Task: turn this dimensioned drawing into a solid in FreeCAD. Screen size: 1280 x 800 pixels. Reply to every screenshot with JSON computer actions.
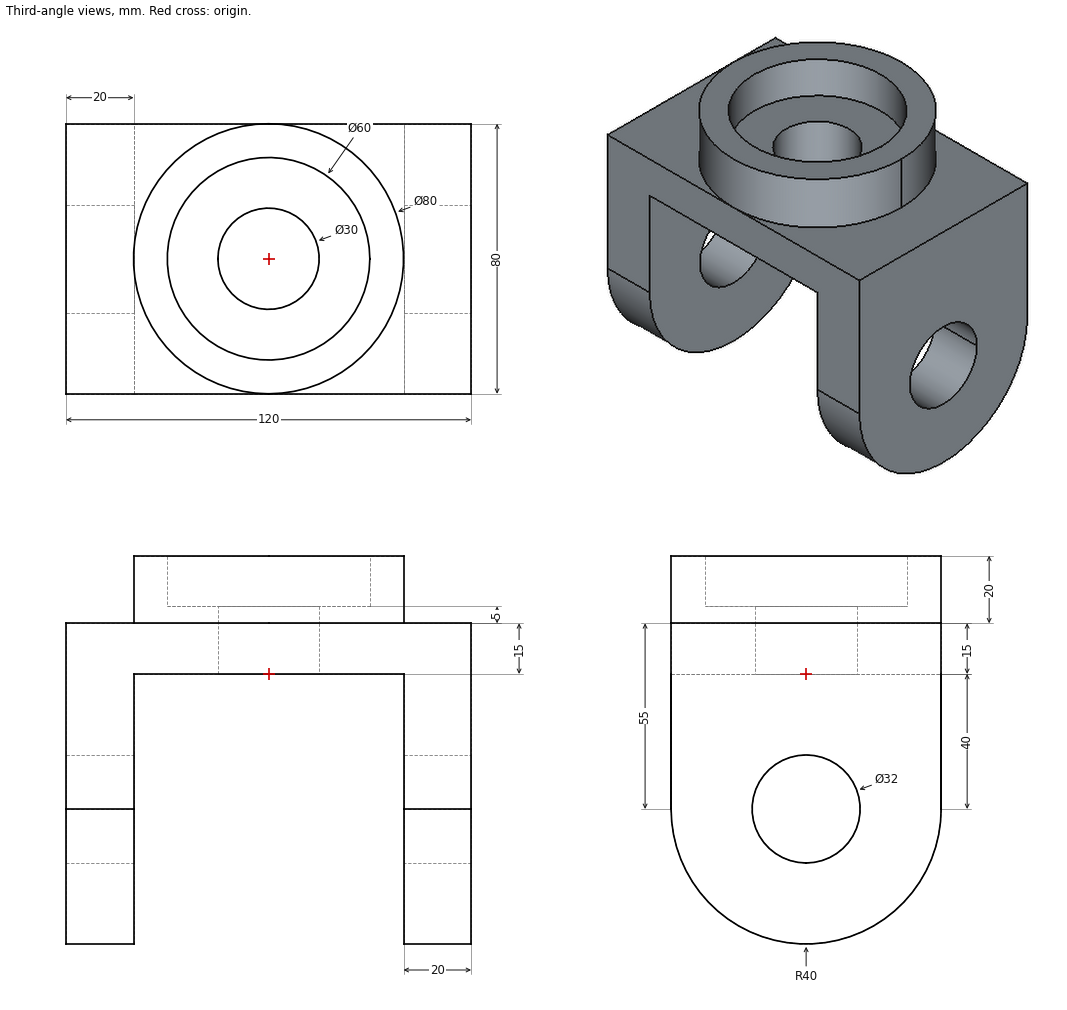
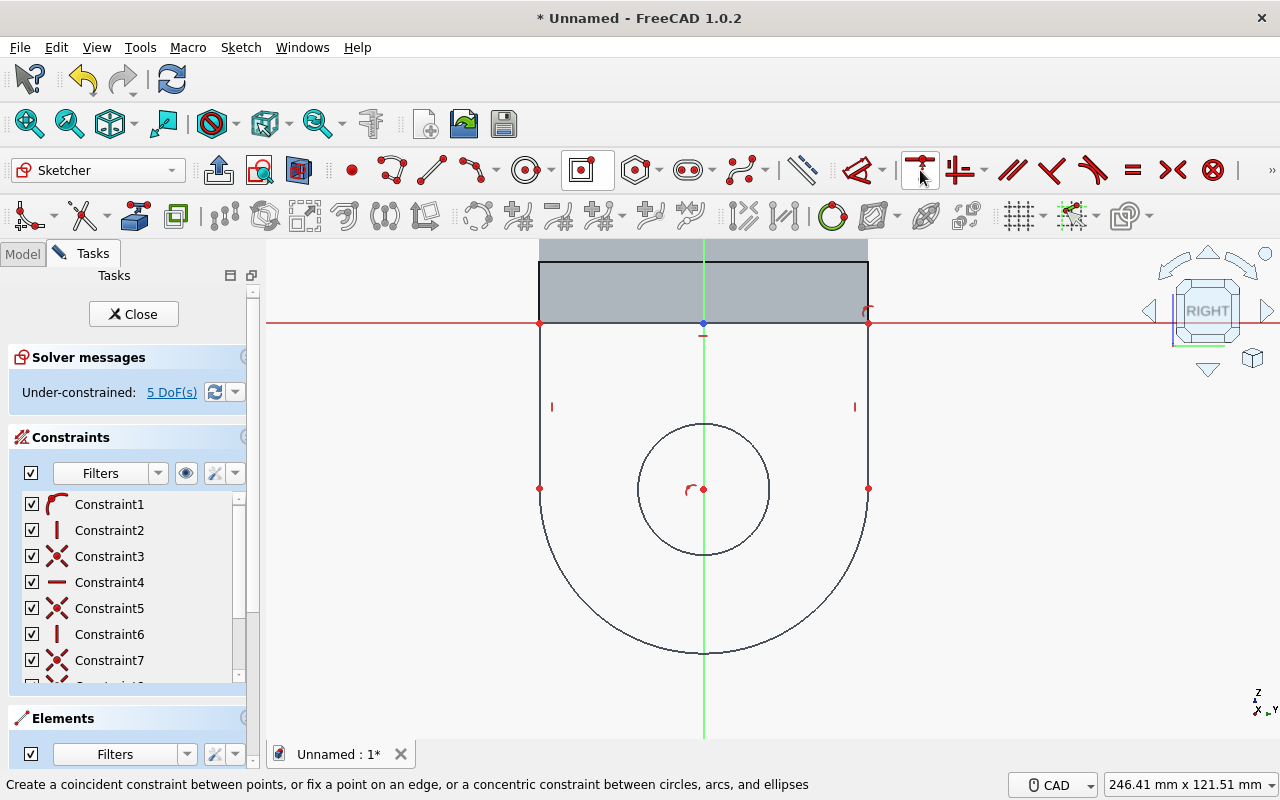
{"action": "left_click", "coordinate": [607, 622]}
{"action": "left_click", "coordinate": [588, 648]}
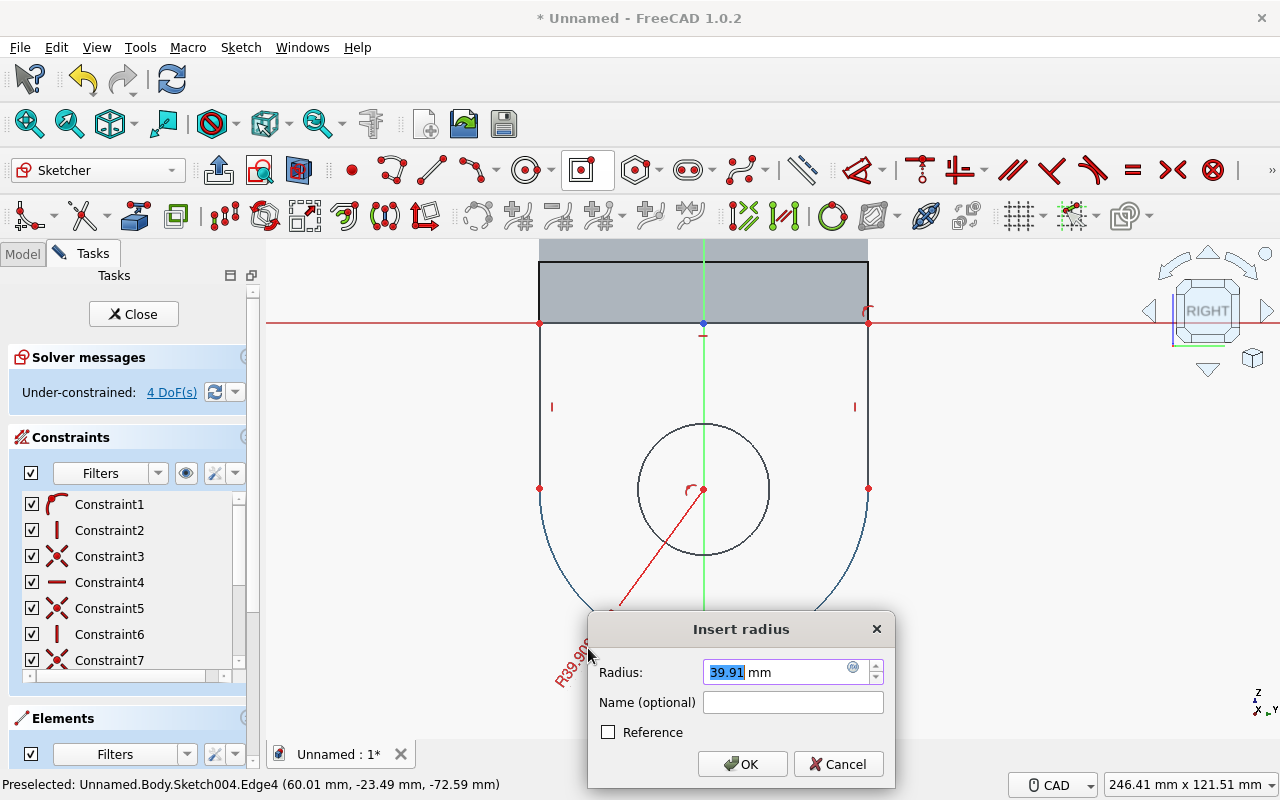
{"action": "type", "text": "40"}
{"action": "key", "text": "Return"}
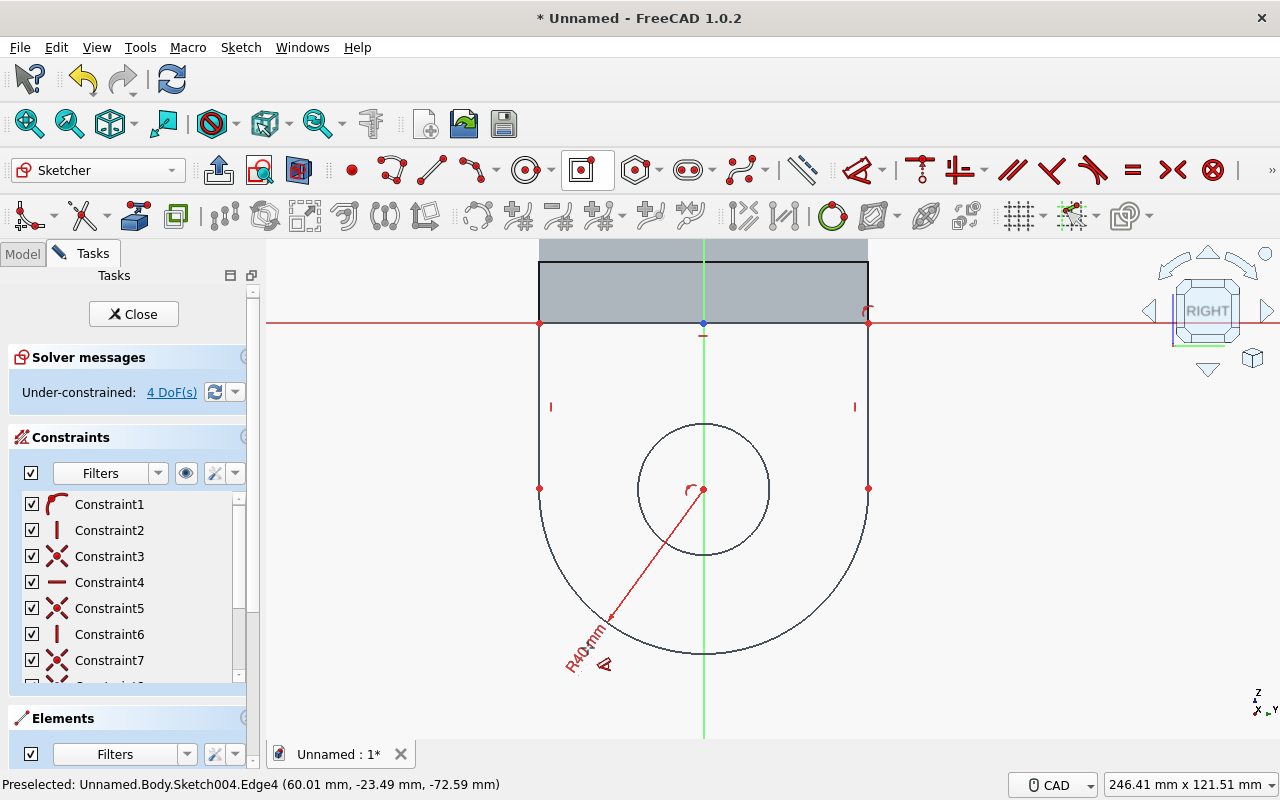
{"action": "left_click", "coordinate": [750, 443]}
{"action": "left_click", "coordinate": [773, 420]}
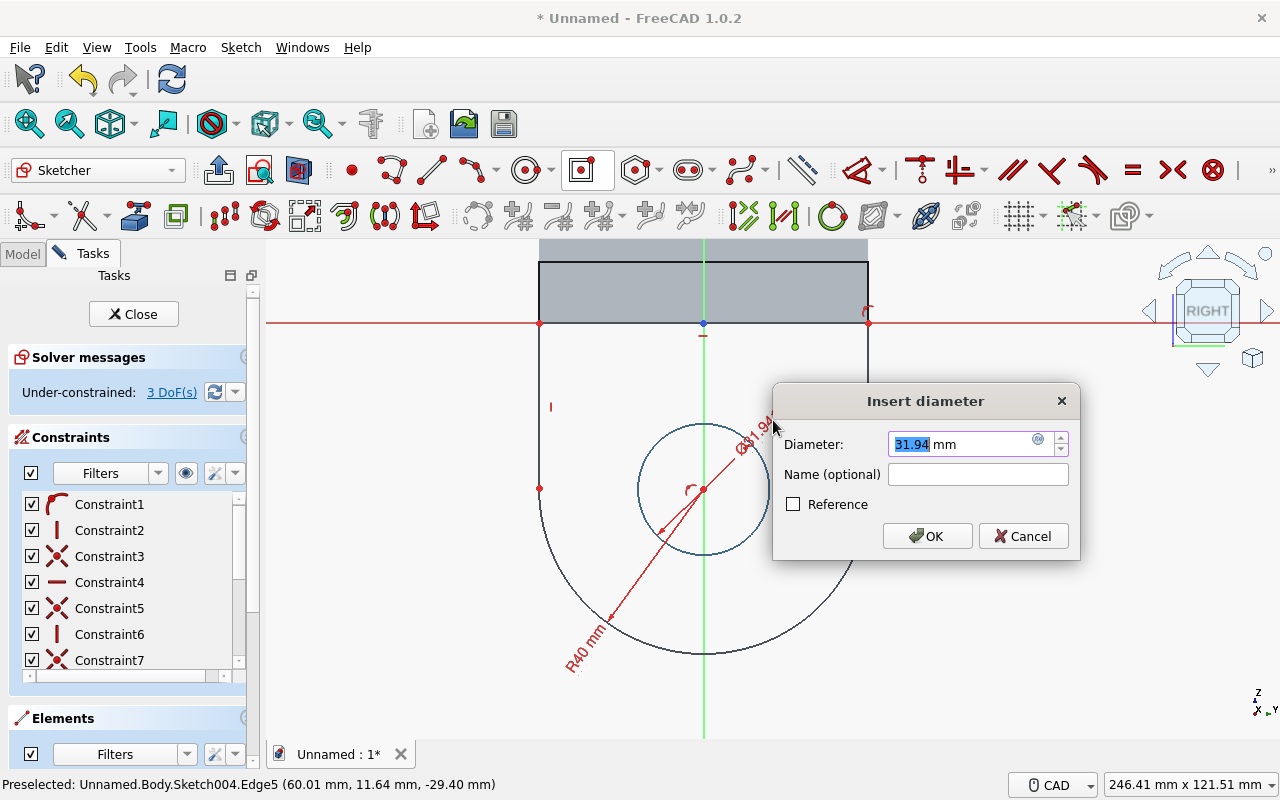
{"action": "type", "text": "32"}
{"action": "key", "text": "Return"}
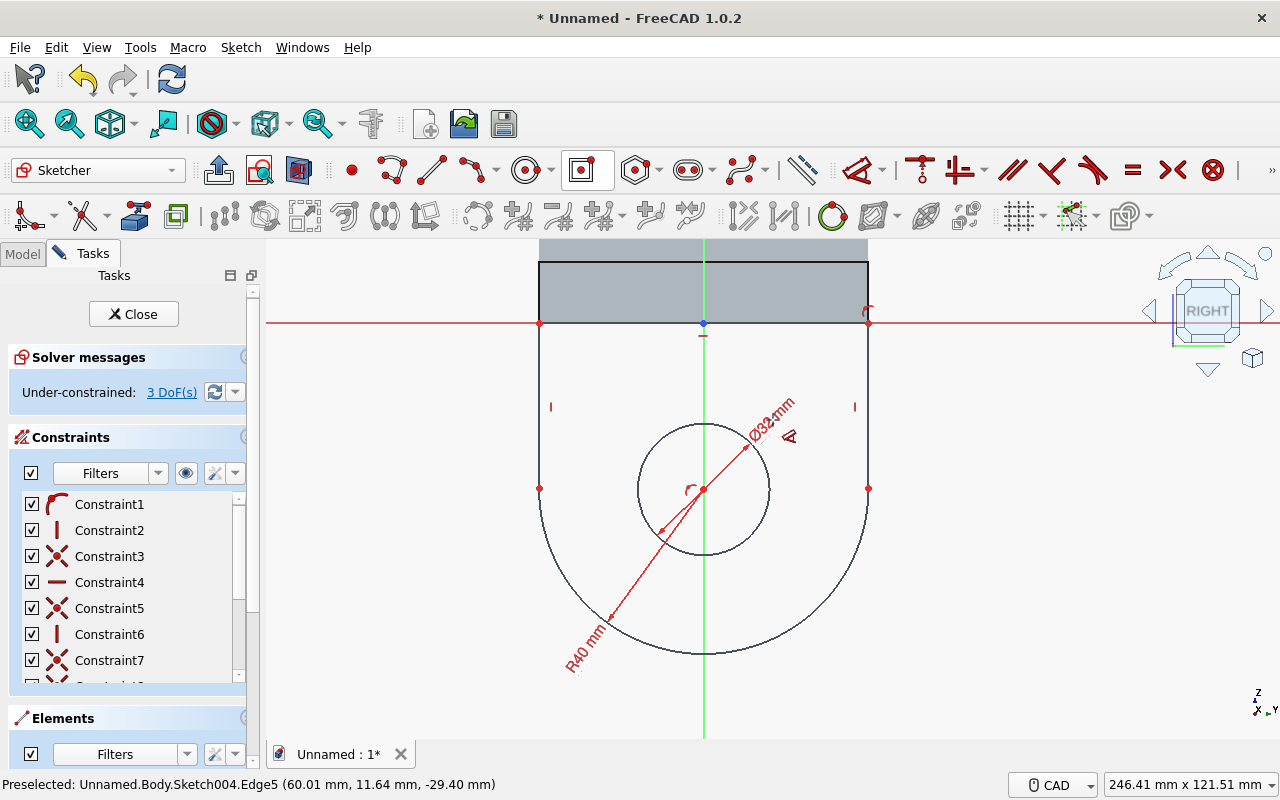
{"action": "left_click", "coordinate": [868, 439]}
{"action": "left_click", "coordinate": [902, 406]}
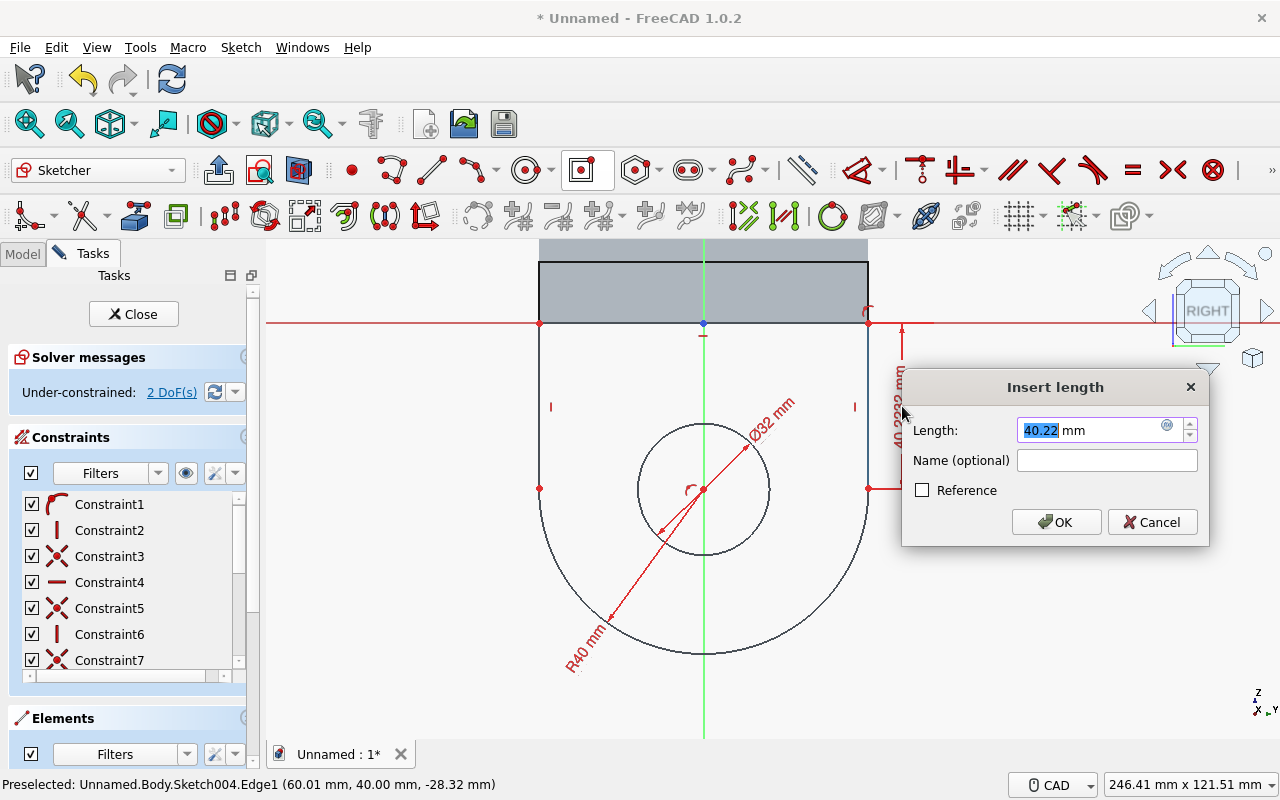
{"action": "type", "text": "40"}
{"action": "key", "text": "Return"}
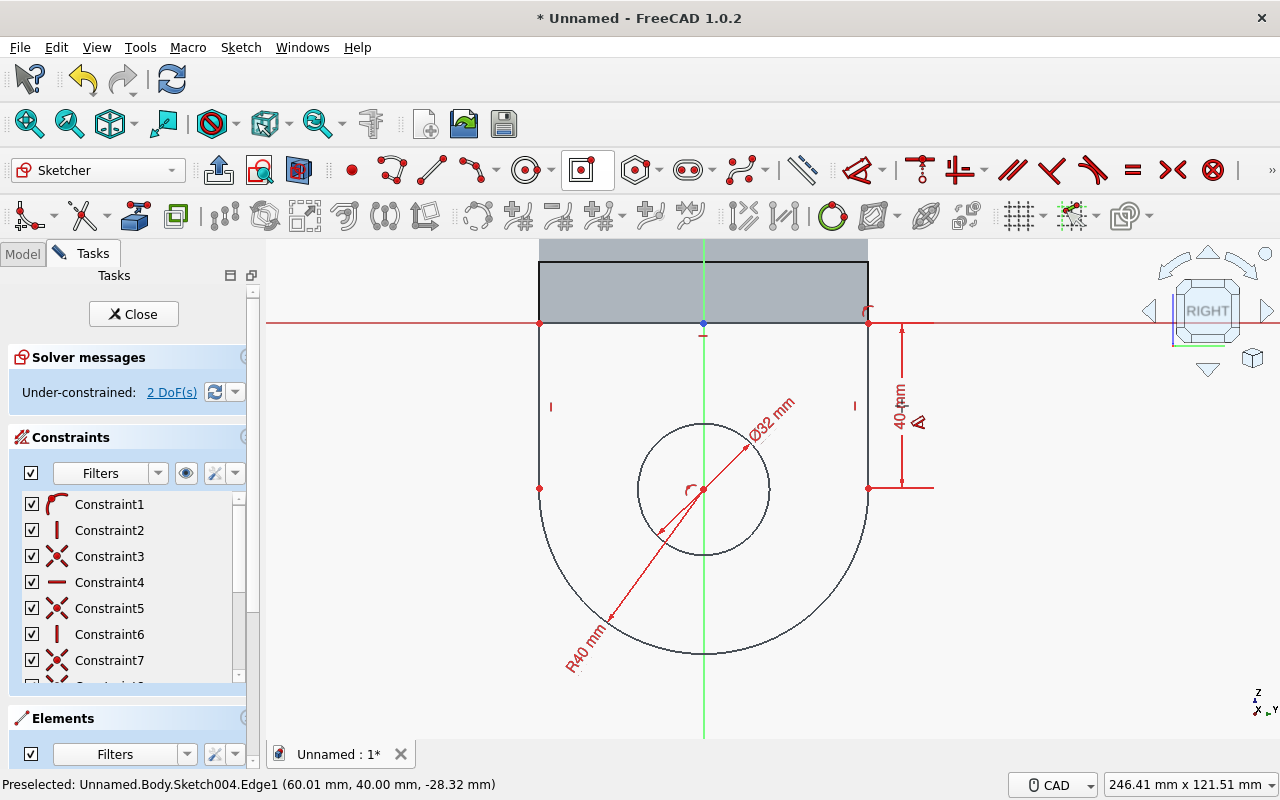
{"action": "left_click", "coordinate": [539, 373]}
{"action": "left_click", "coordinate": [505, 406]}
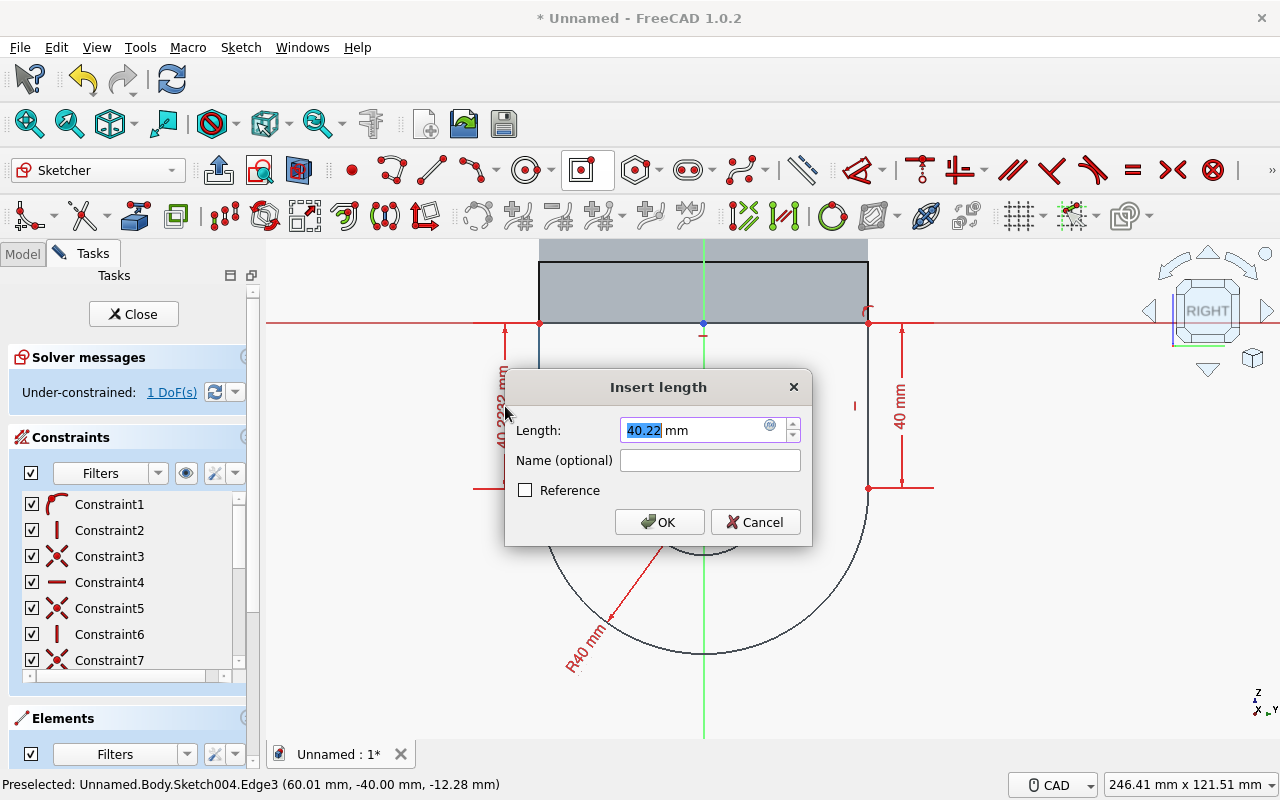
{"action": "type", "text": "40"}
{"action": "key", "text": "Return"}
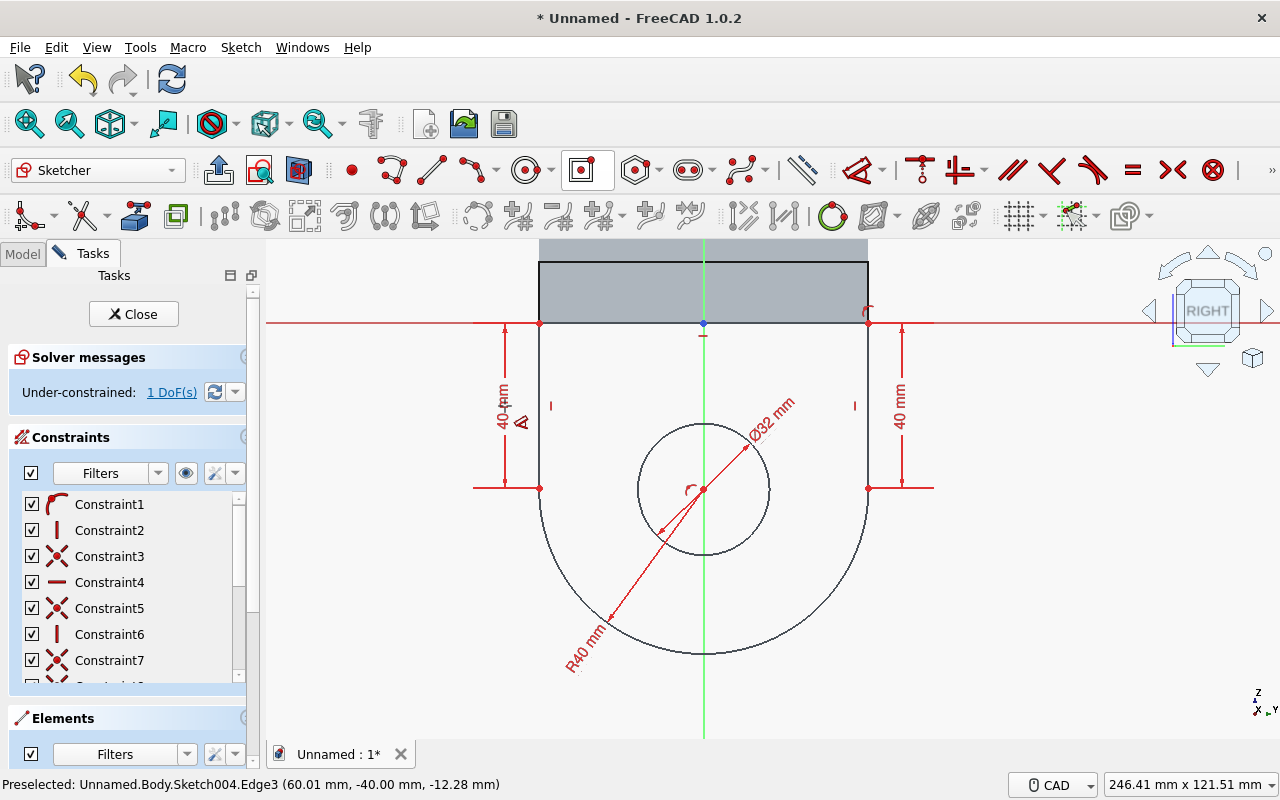
{"action": "left_click", "coordinate": [704, 489]}
{"action": "left_click", "coordinate": [738, 368]}